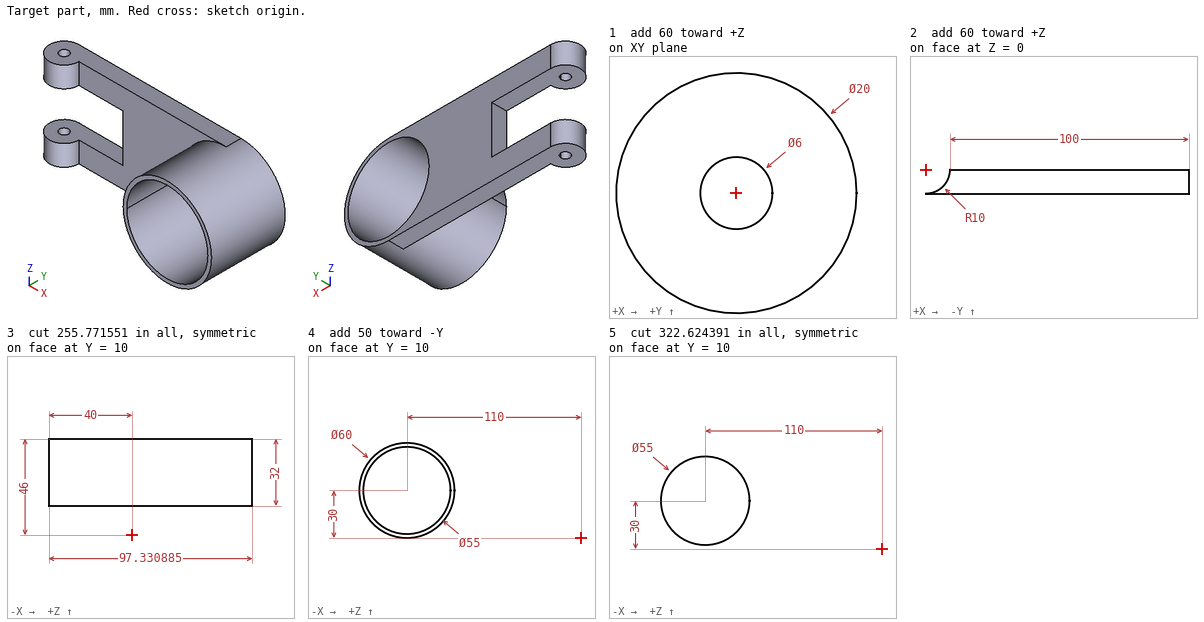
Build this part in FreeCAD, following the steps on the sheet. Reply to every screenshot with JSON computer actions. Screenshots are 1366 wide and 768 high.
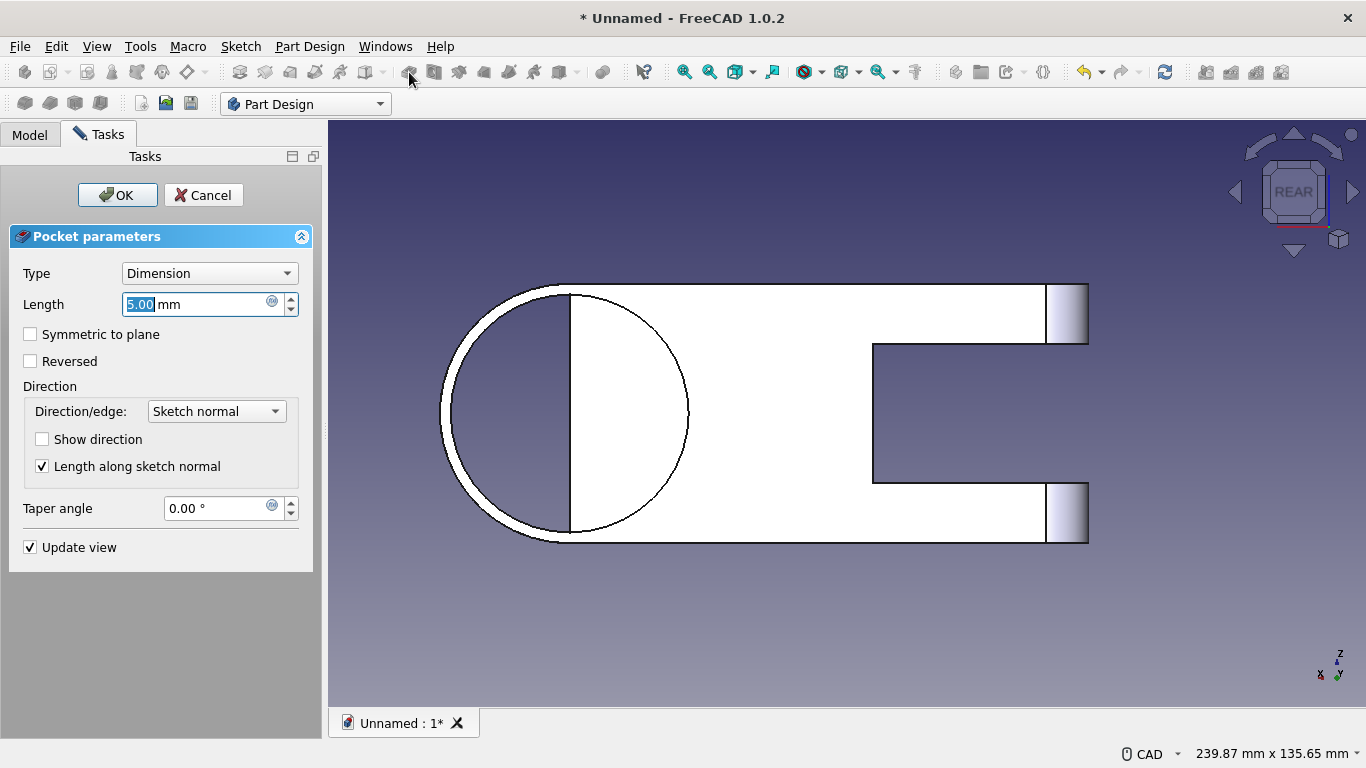
{"action": "type", "text": "322.624391"}
{"action": "key", "text": "Tab"}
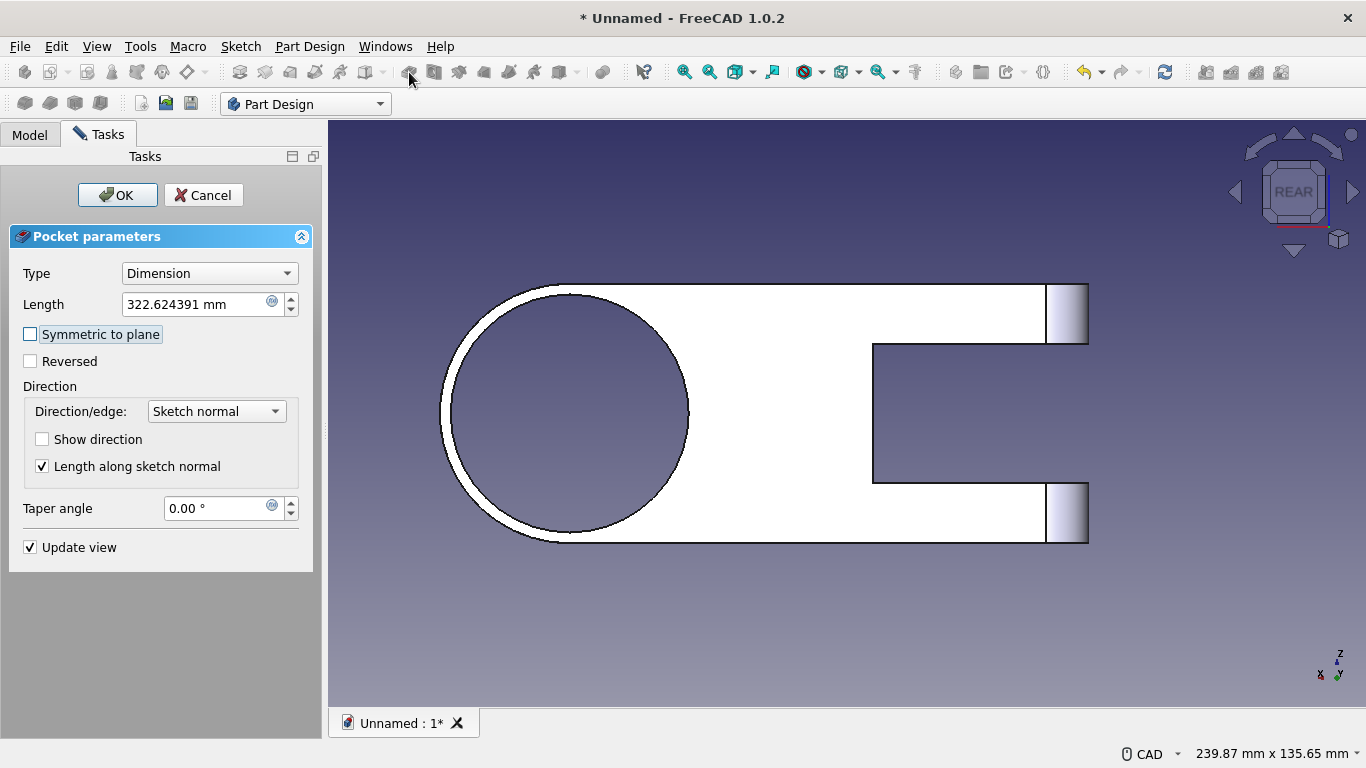
{"action": "left_click", "coordinate": [31, 334]}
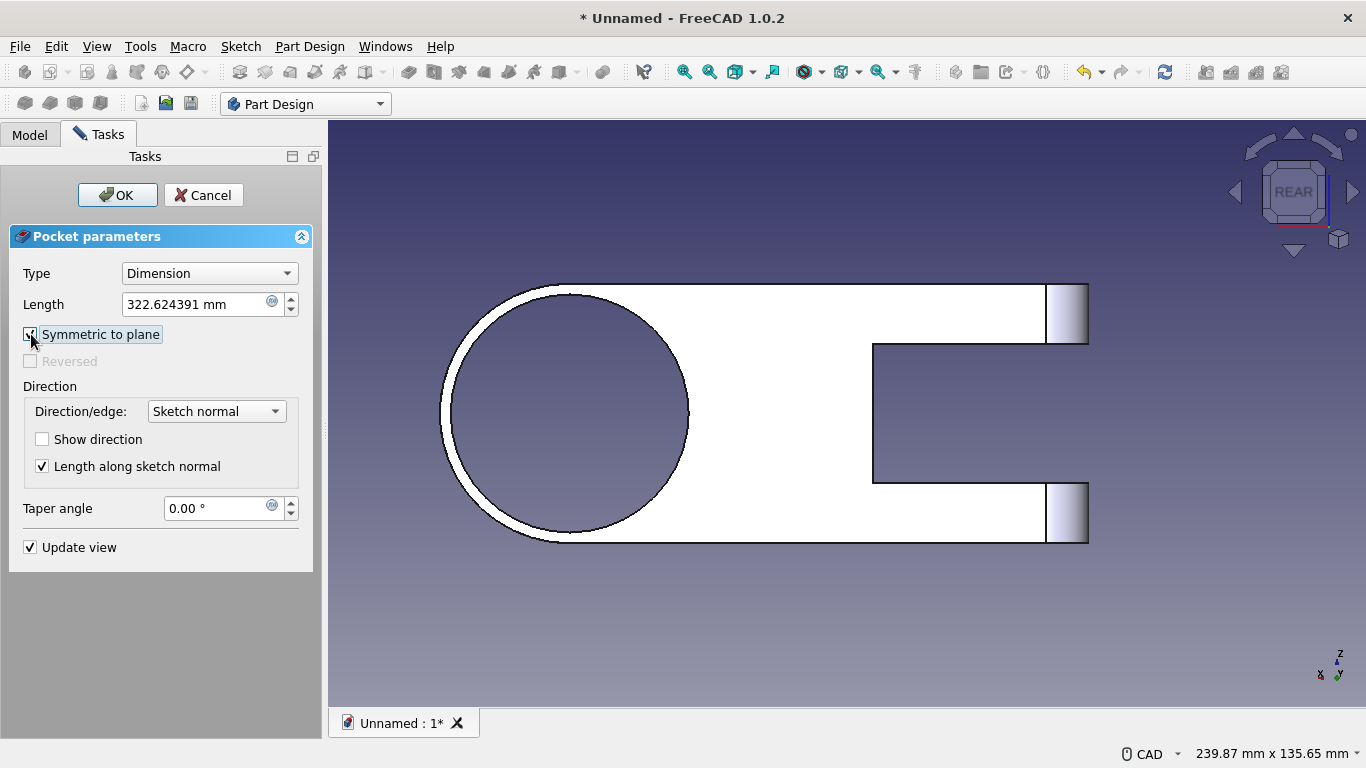
{"action": "left_click", "coordinate": [118, 195]}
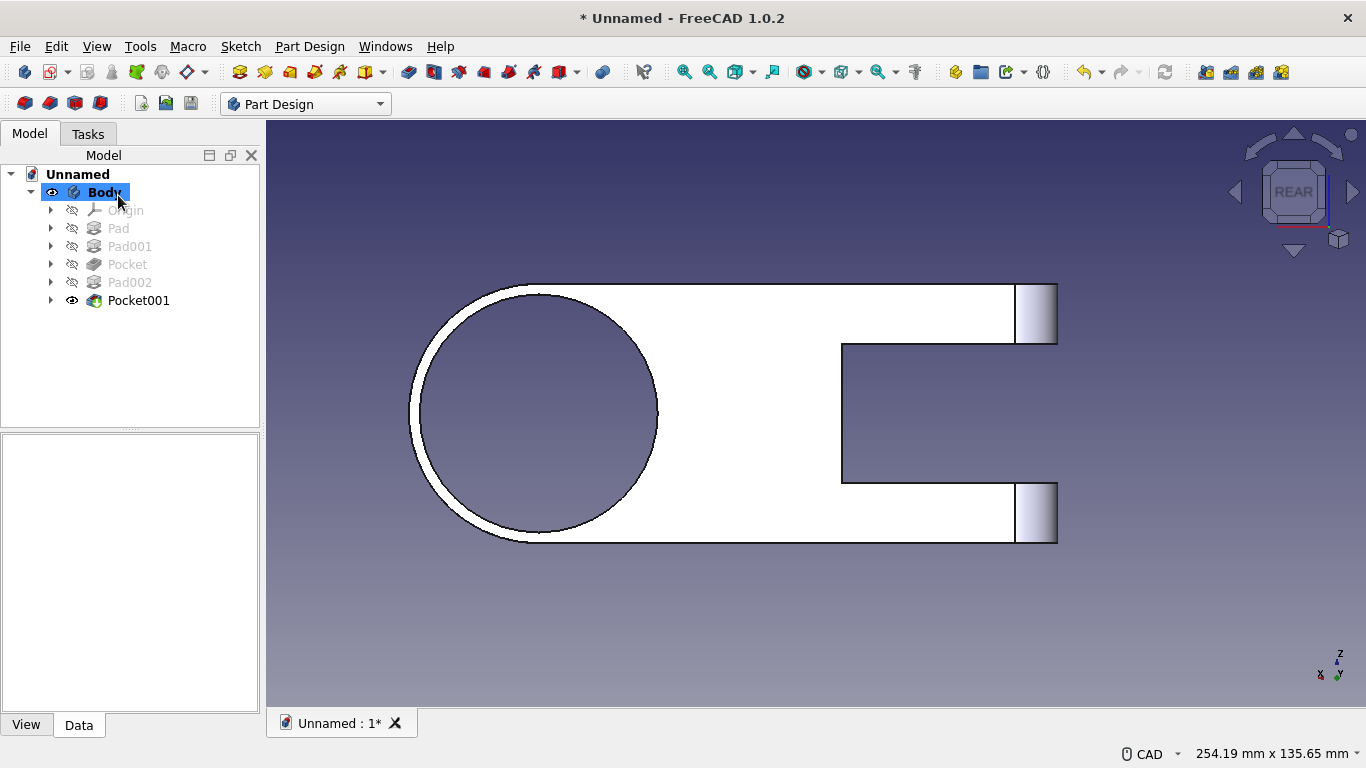
{"action": "key", "text": "0"}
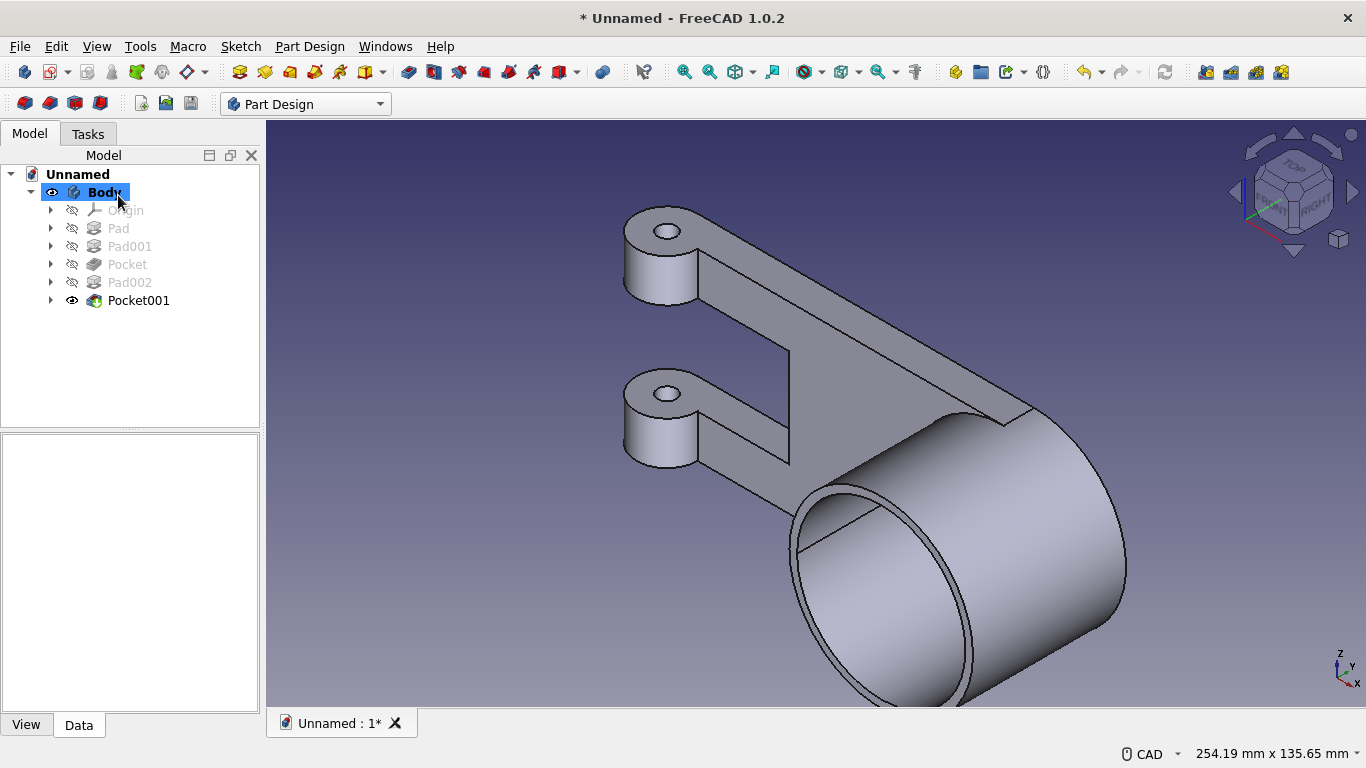
{"action": "left_click", "coordinate": [685, 72]}